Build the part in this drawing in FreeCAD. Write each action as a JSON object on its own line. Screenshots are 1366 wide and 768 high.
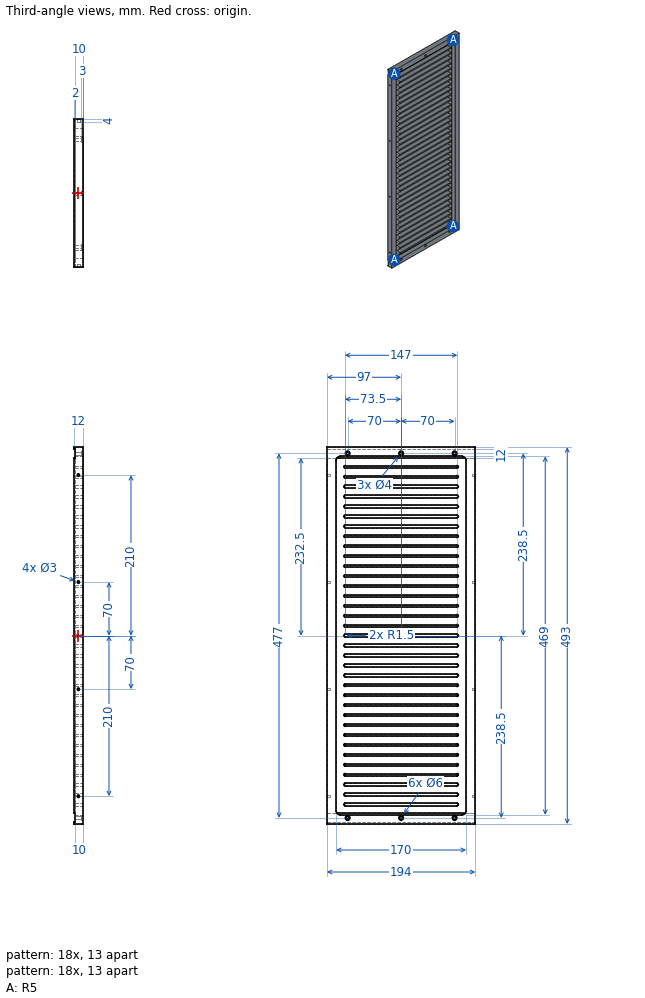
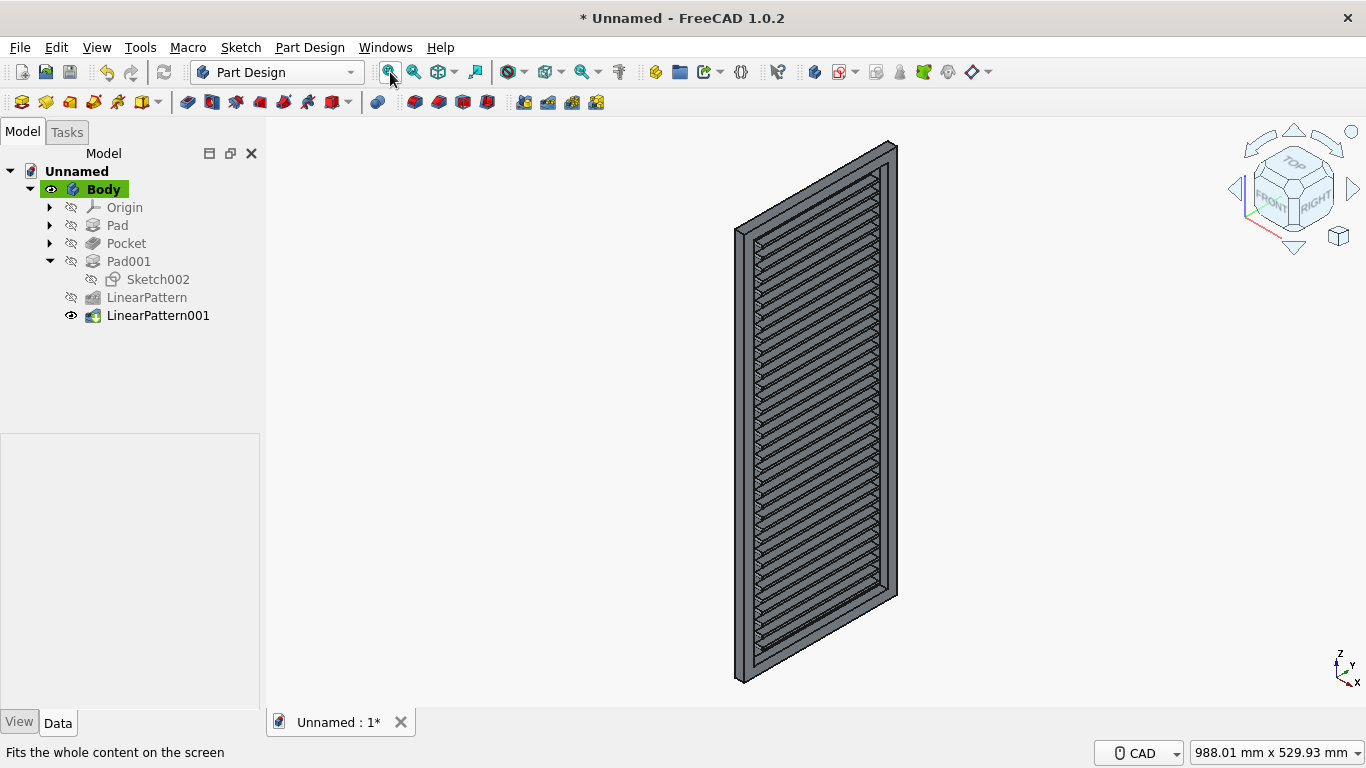
{"action": "scroll", "coordinate": [750, 663], "scroll_direction": "up", "scroll_amount": 7}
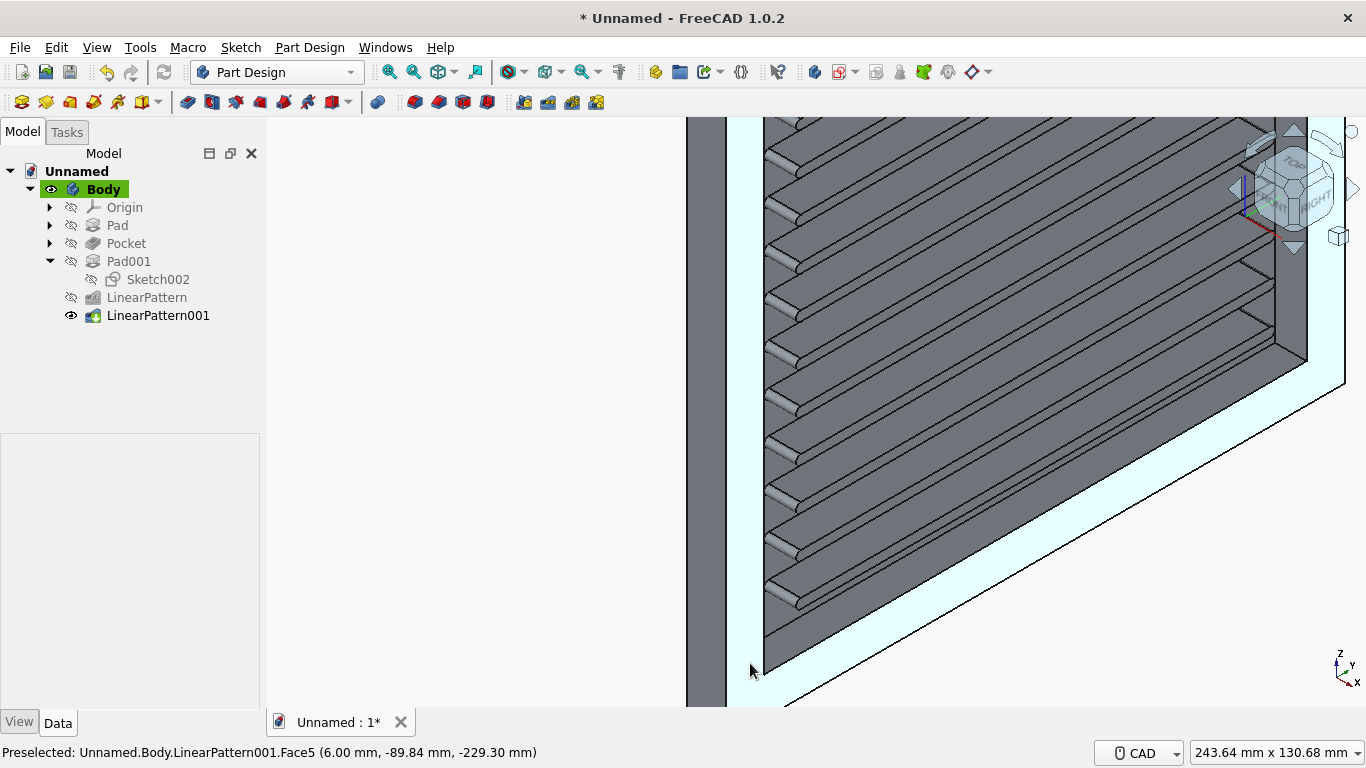
{"action": "left_click", "coordinate": [390, 72]}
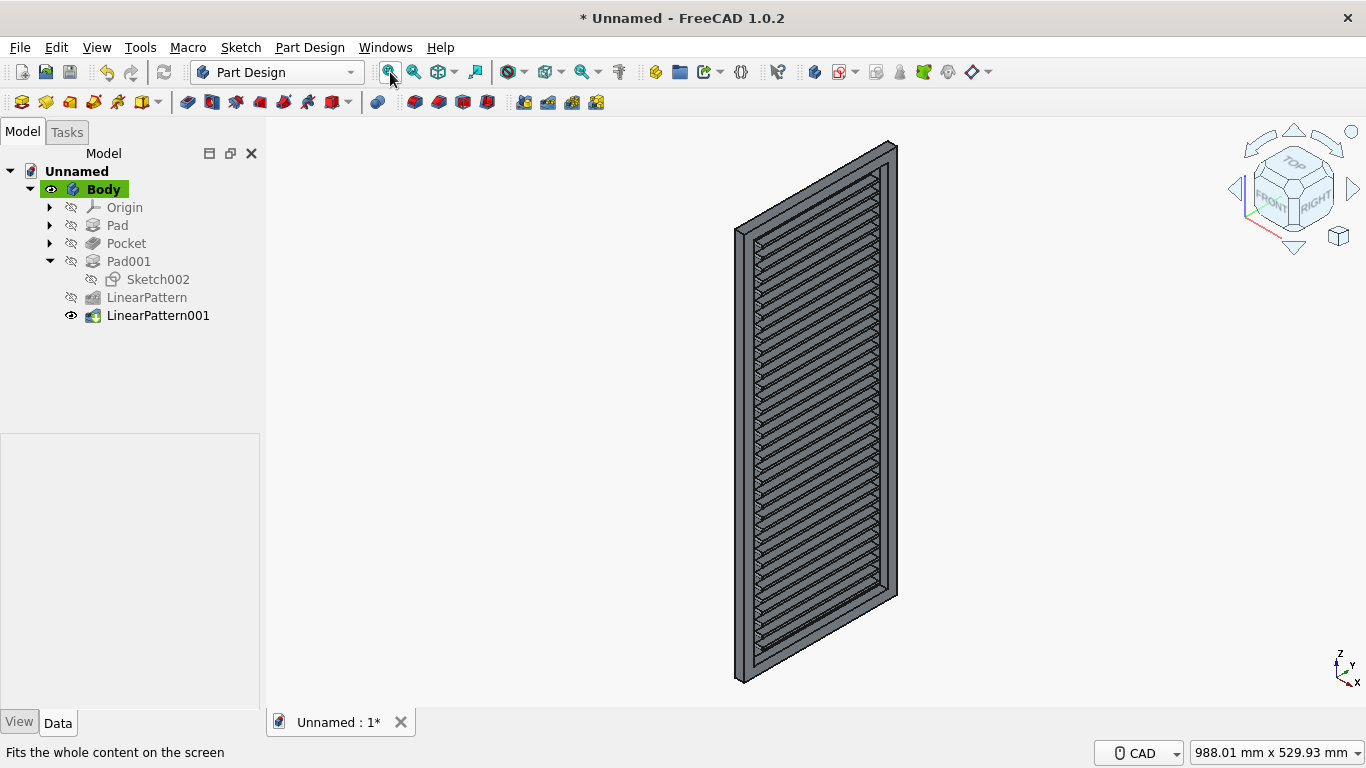
{"action": "key", "text": "2"}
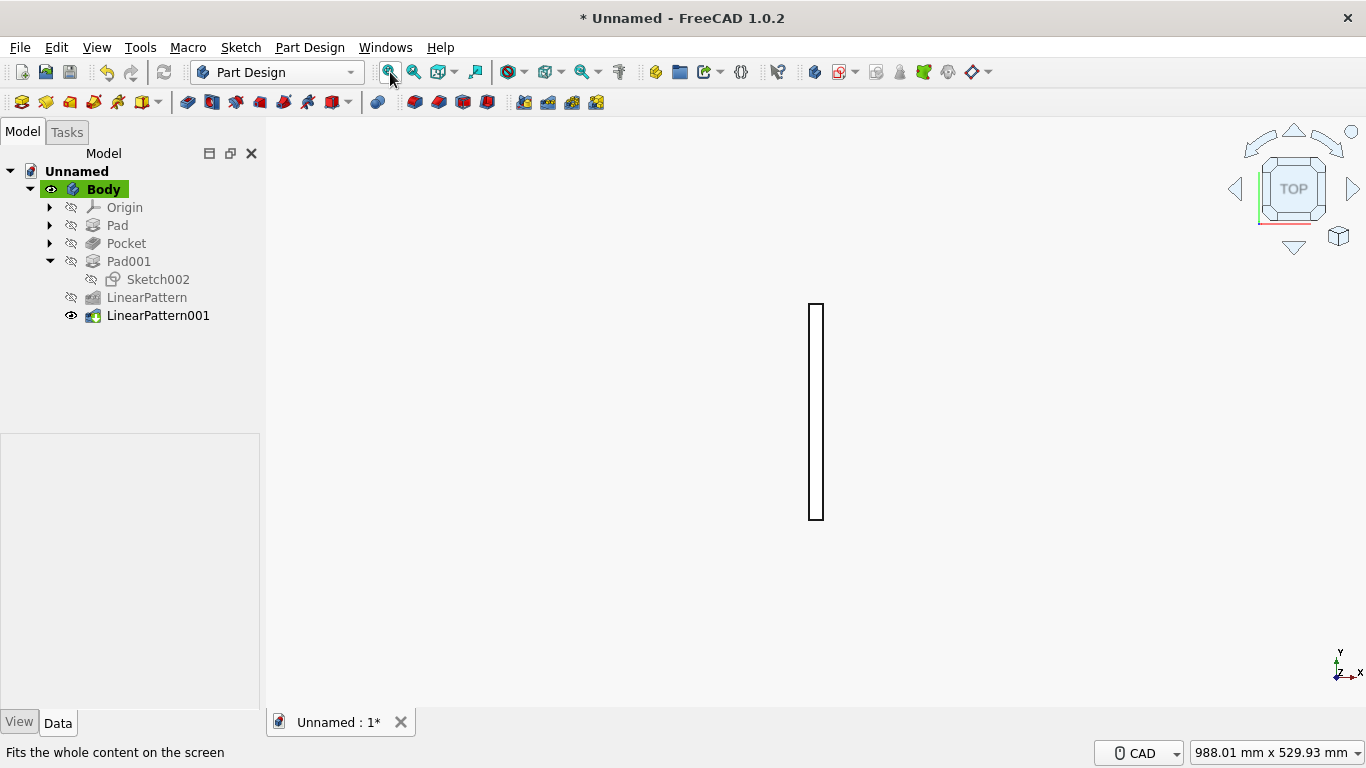
{"action": "left_click", "coordinate": [390, 72]}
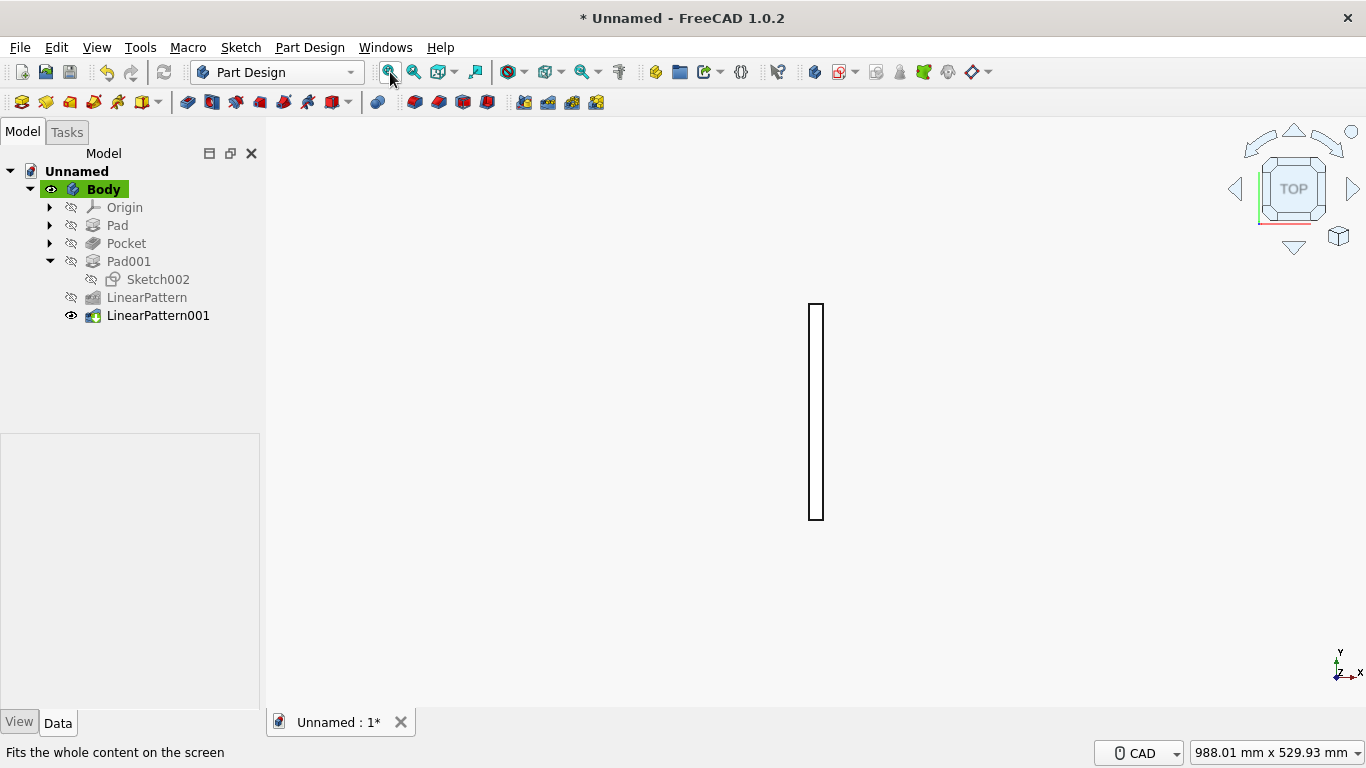
{"action": "scroll", "coordinate": [817, 506], "scroll_direction": "up", "scroll_amount": 7}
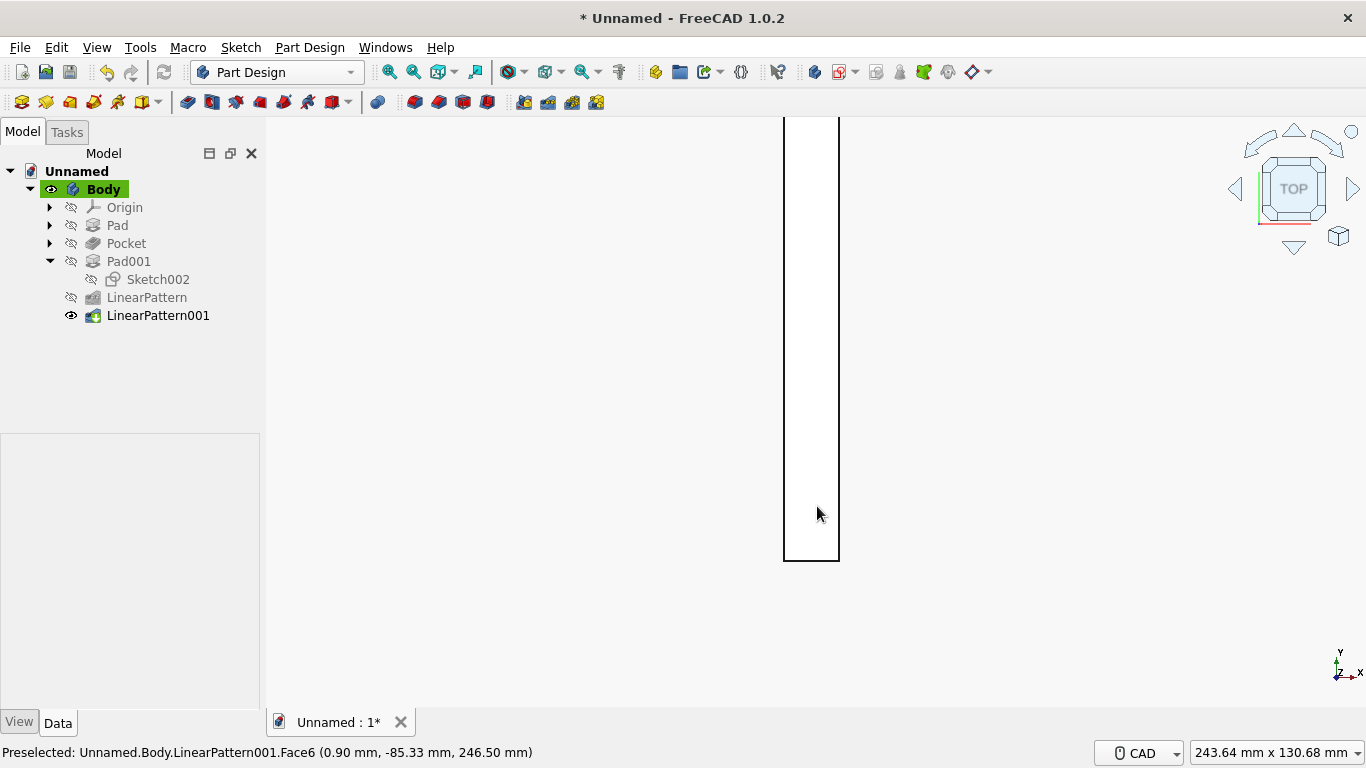
{"action": "key", "text": "v f"}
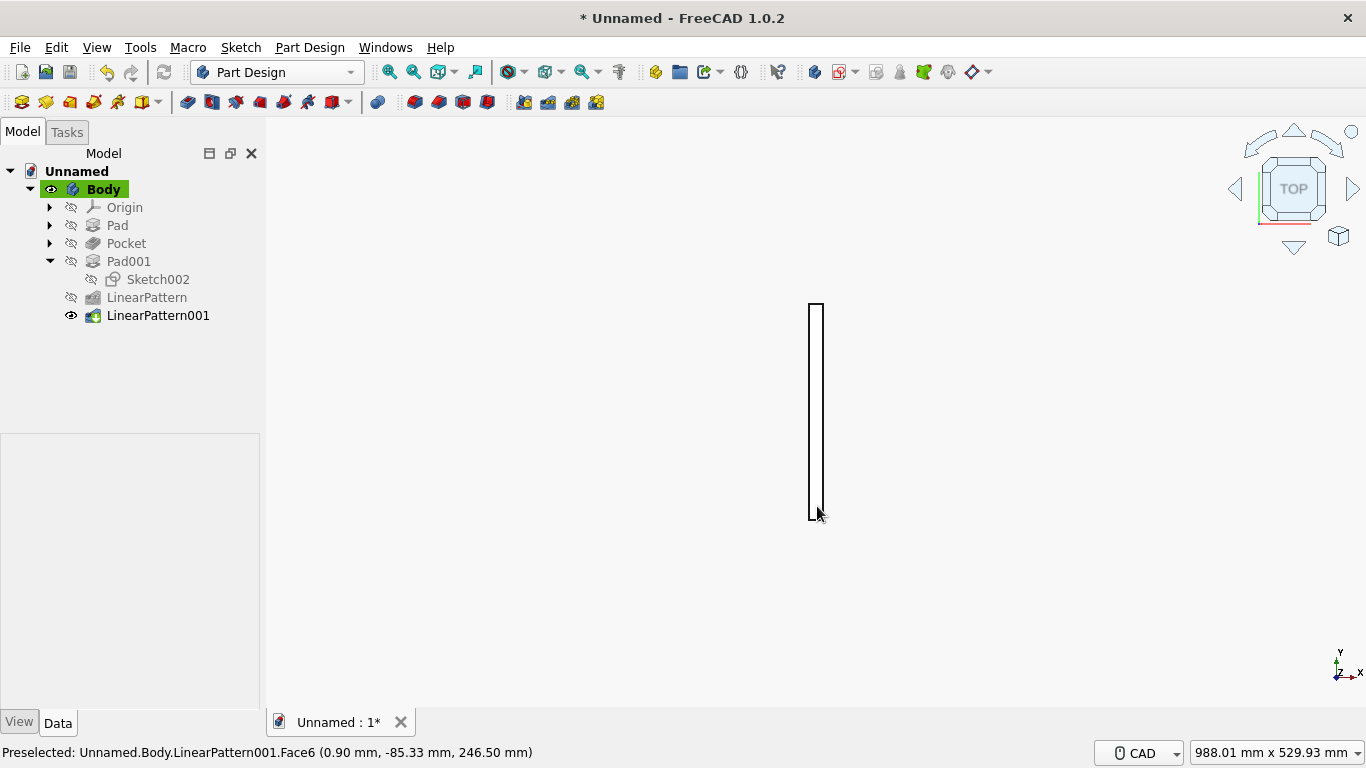
{"action": "key", "text": "1"}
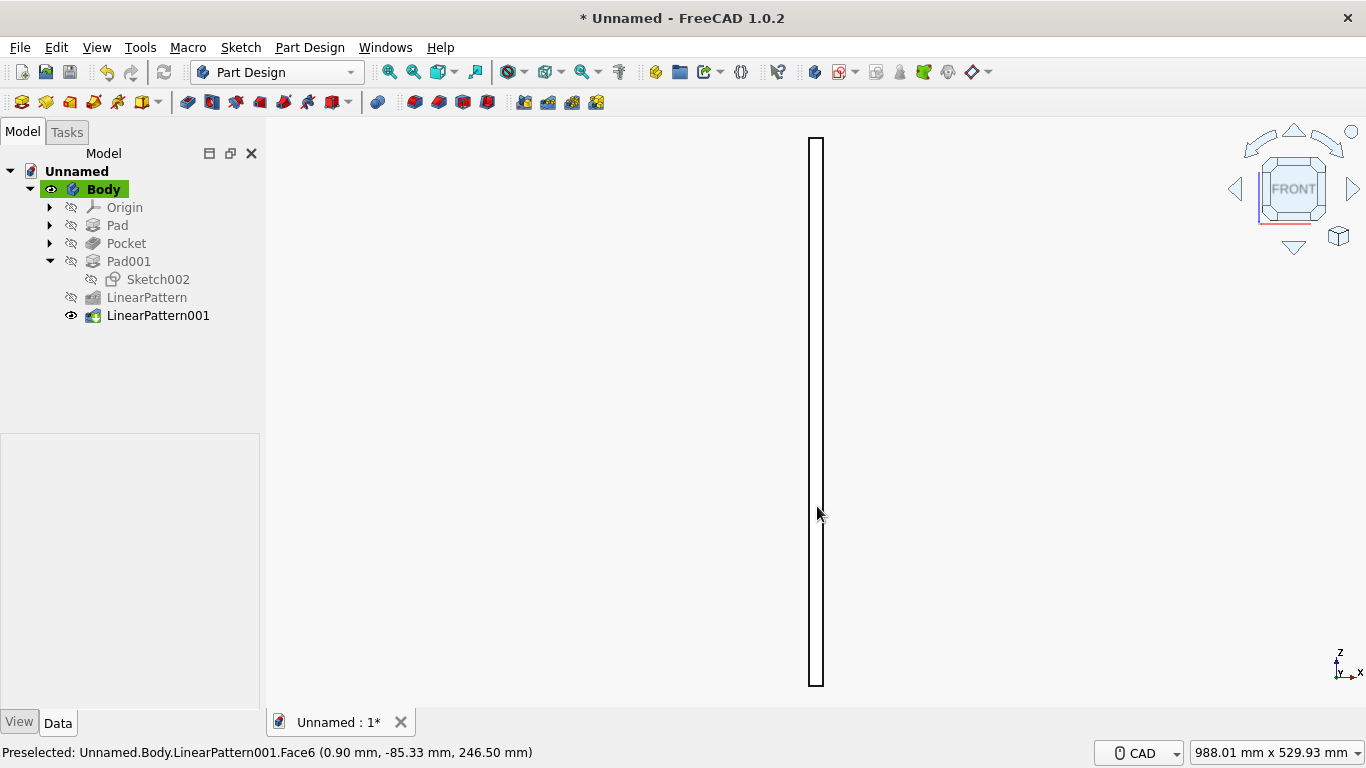
{"action": "scroll", "coordinate": [817, 672], "scroll_direction": "up", "scroll_amount": 7}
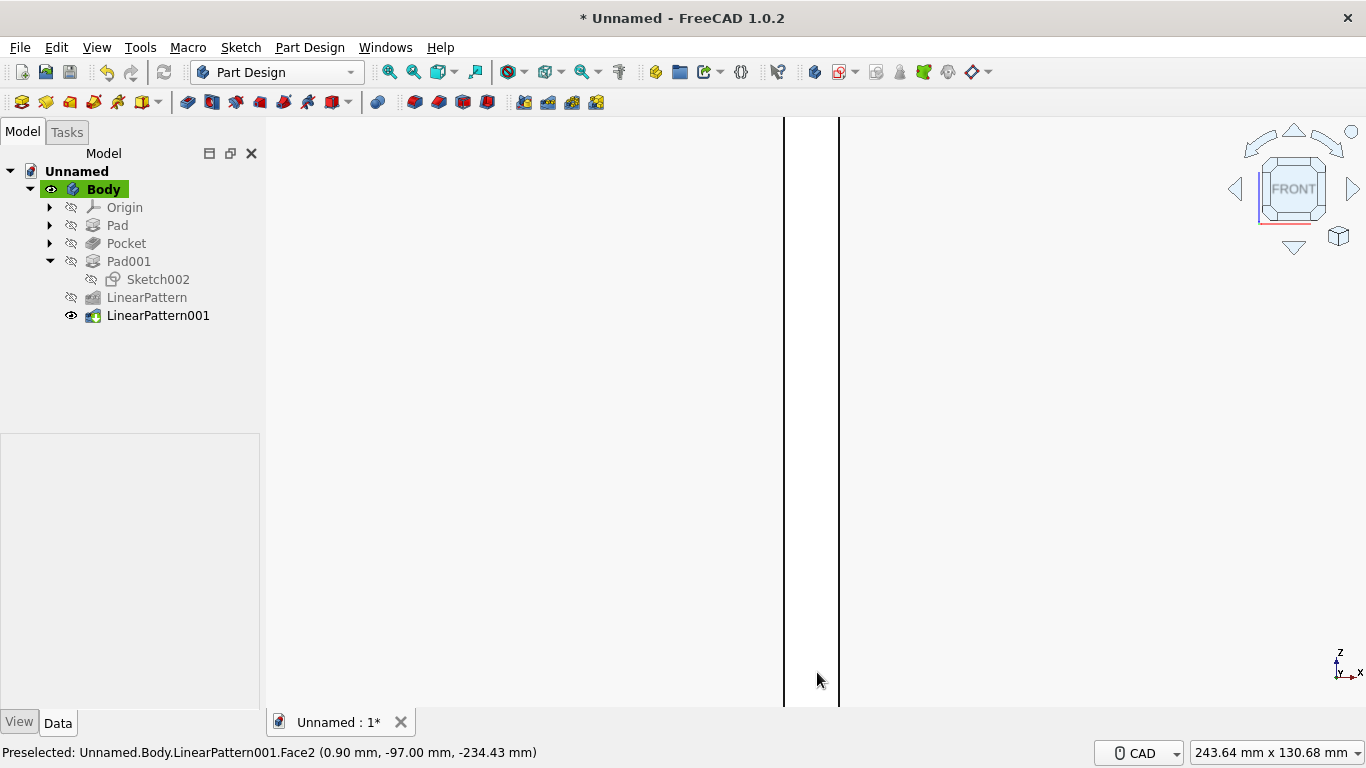
{"action": "left_click", "coordinate": [390, 72]}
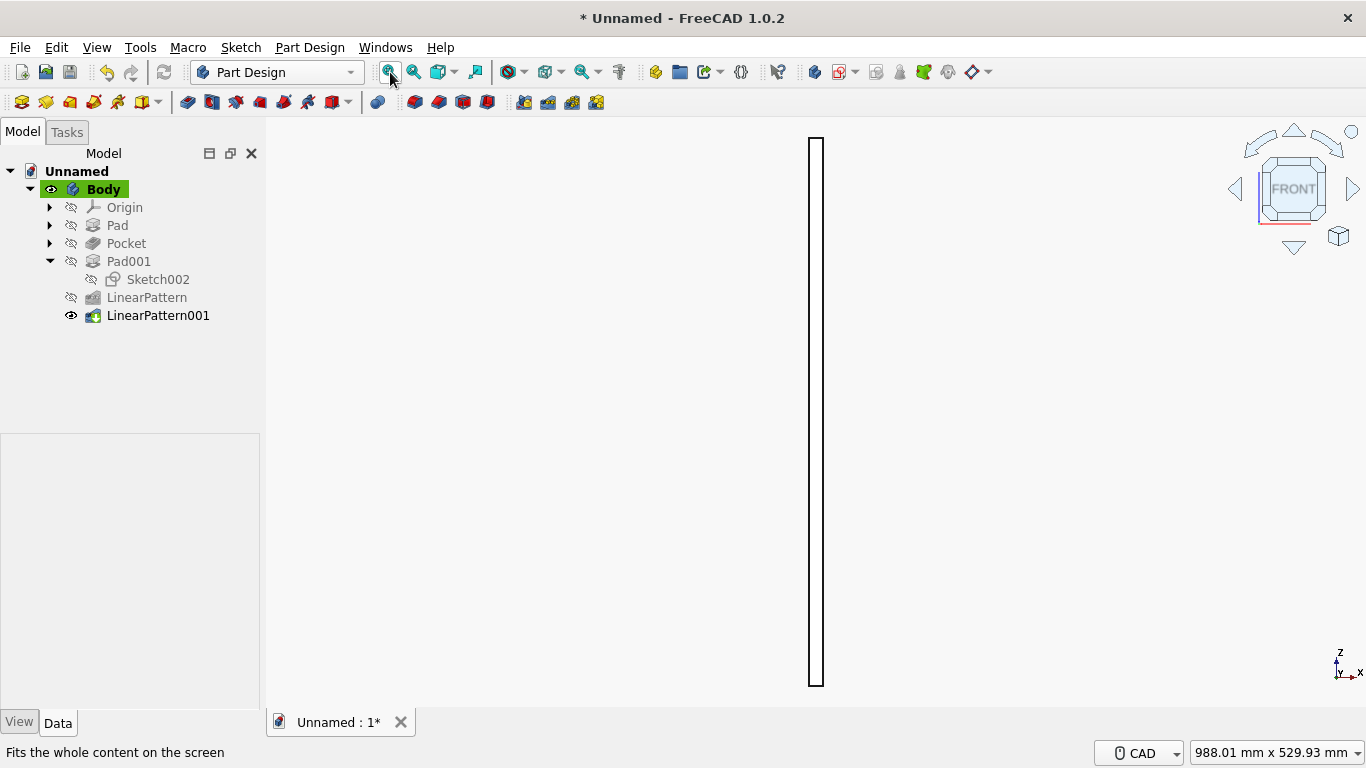
{"action": "key", "text": "3"}